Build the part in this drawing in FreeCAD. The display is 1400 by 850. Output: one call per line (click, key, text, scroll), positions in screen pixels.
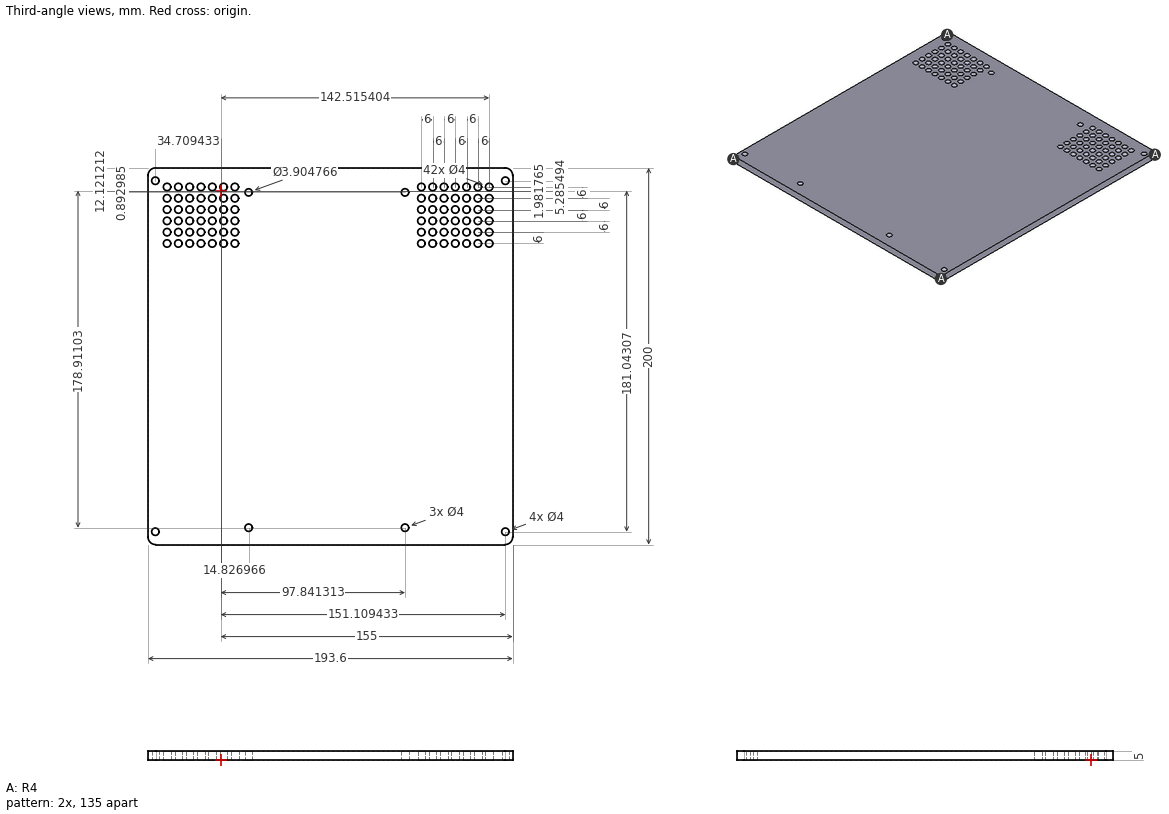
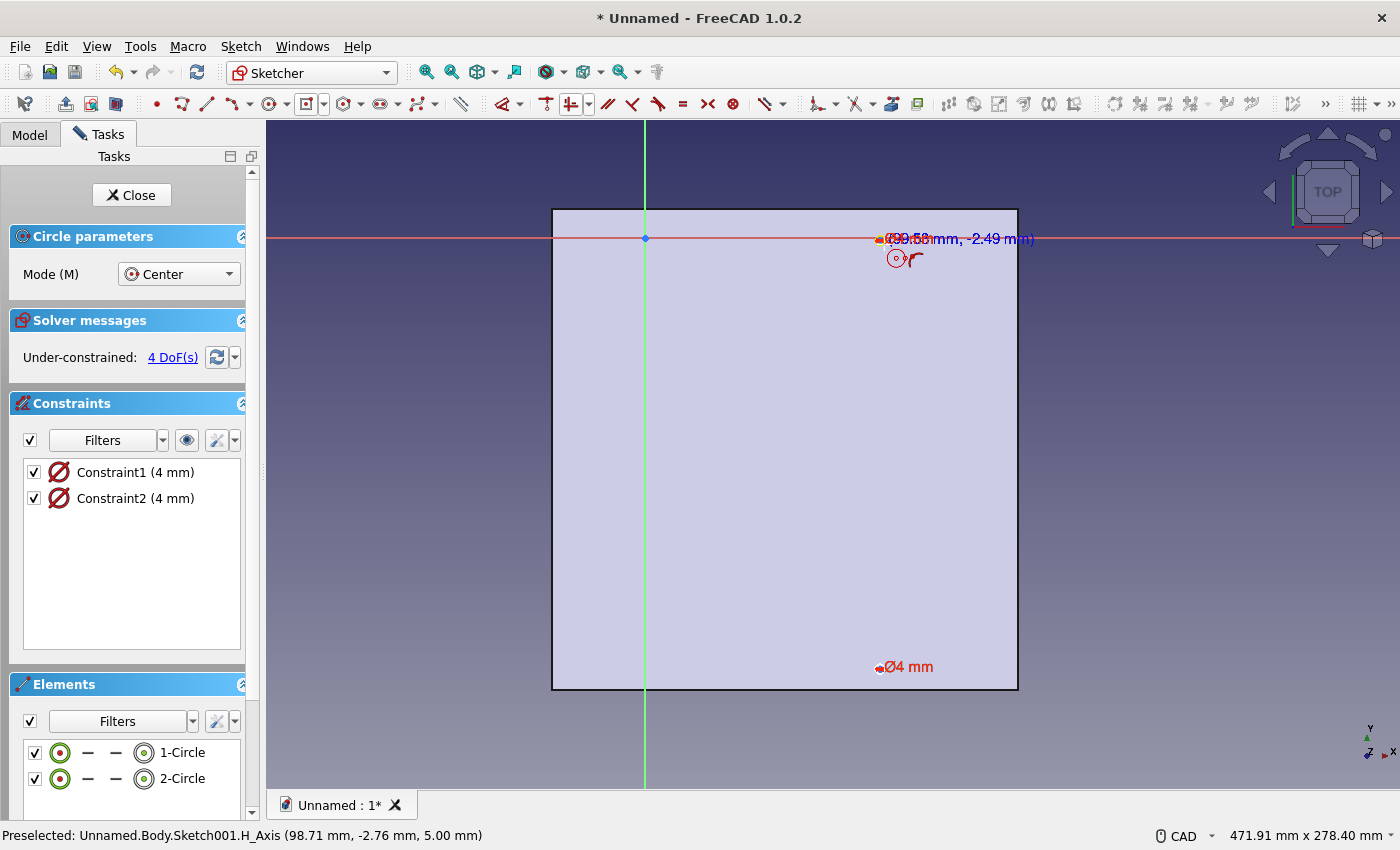
scroll(681, 668, up, 8)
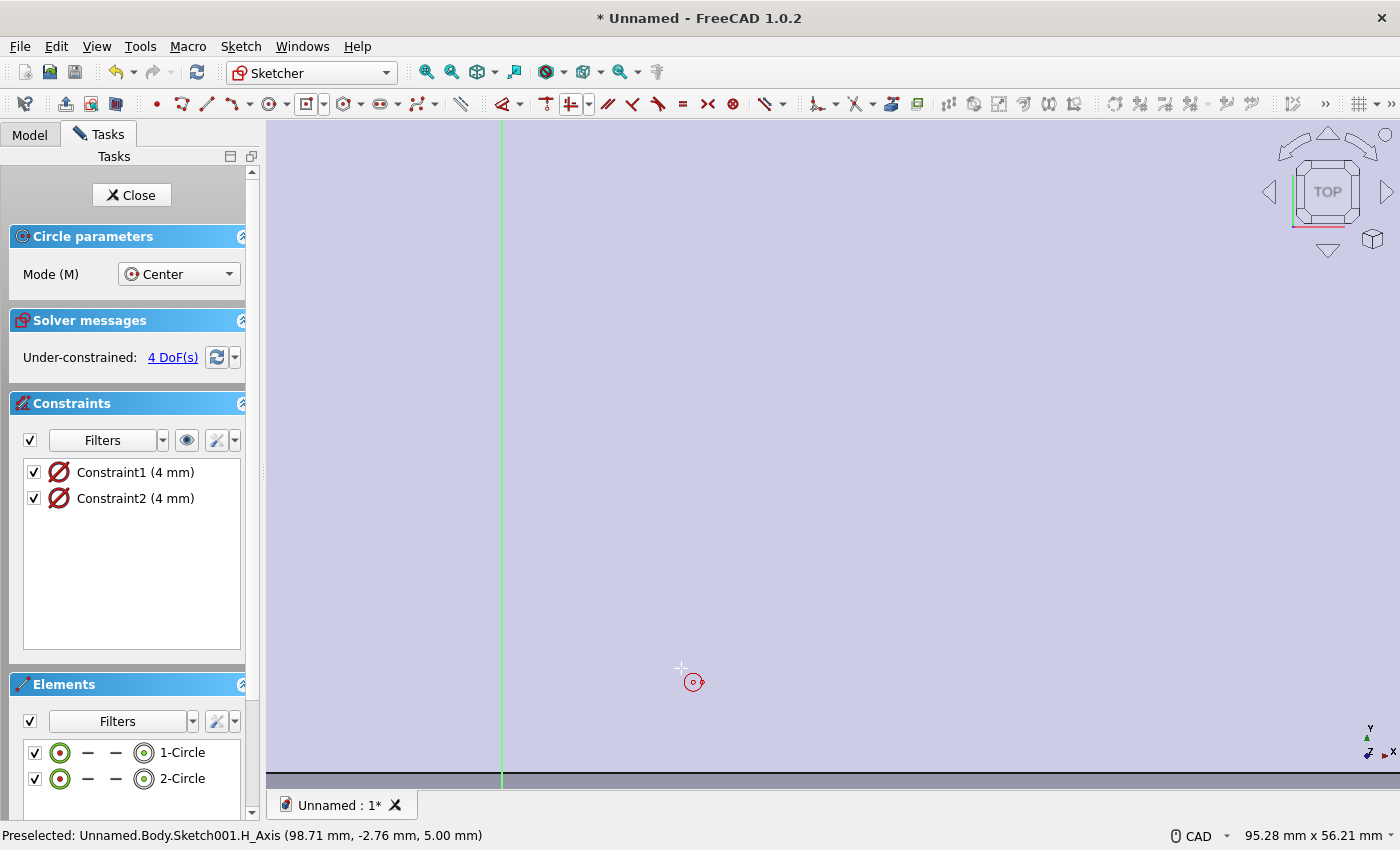
scroll(681, 669, down, 8)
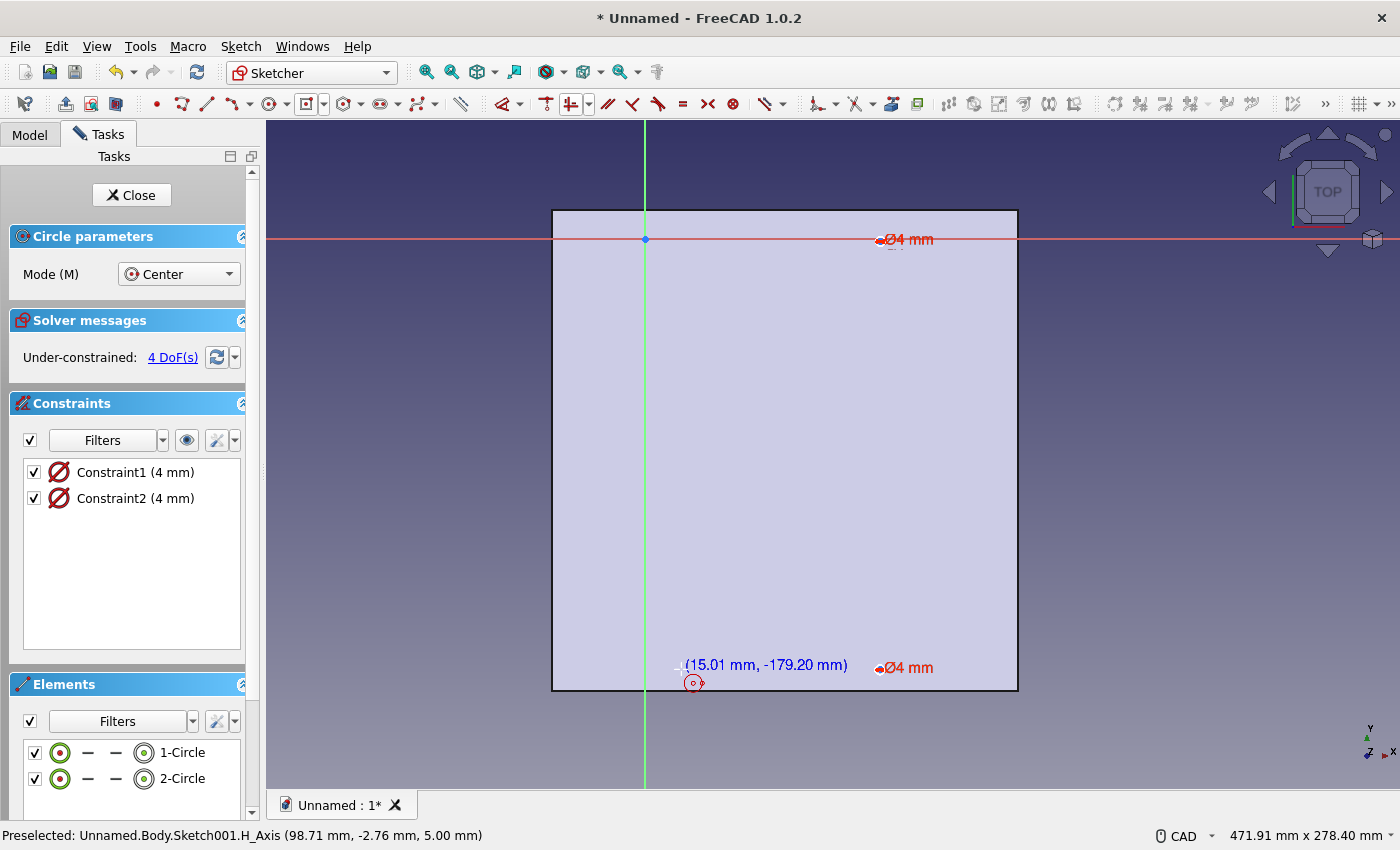
click(681, 669)
move(684, 666)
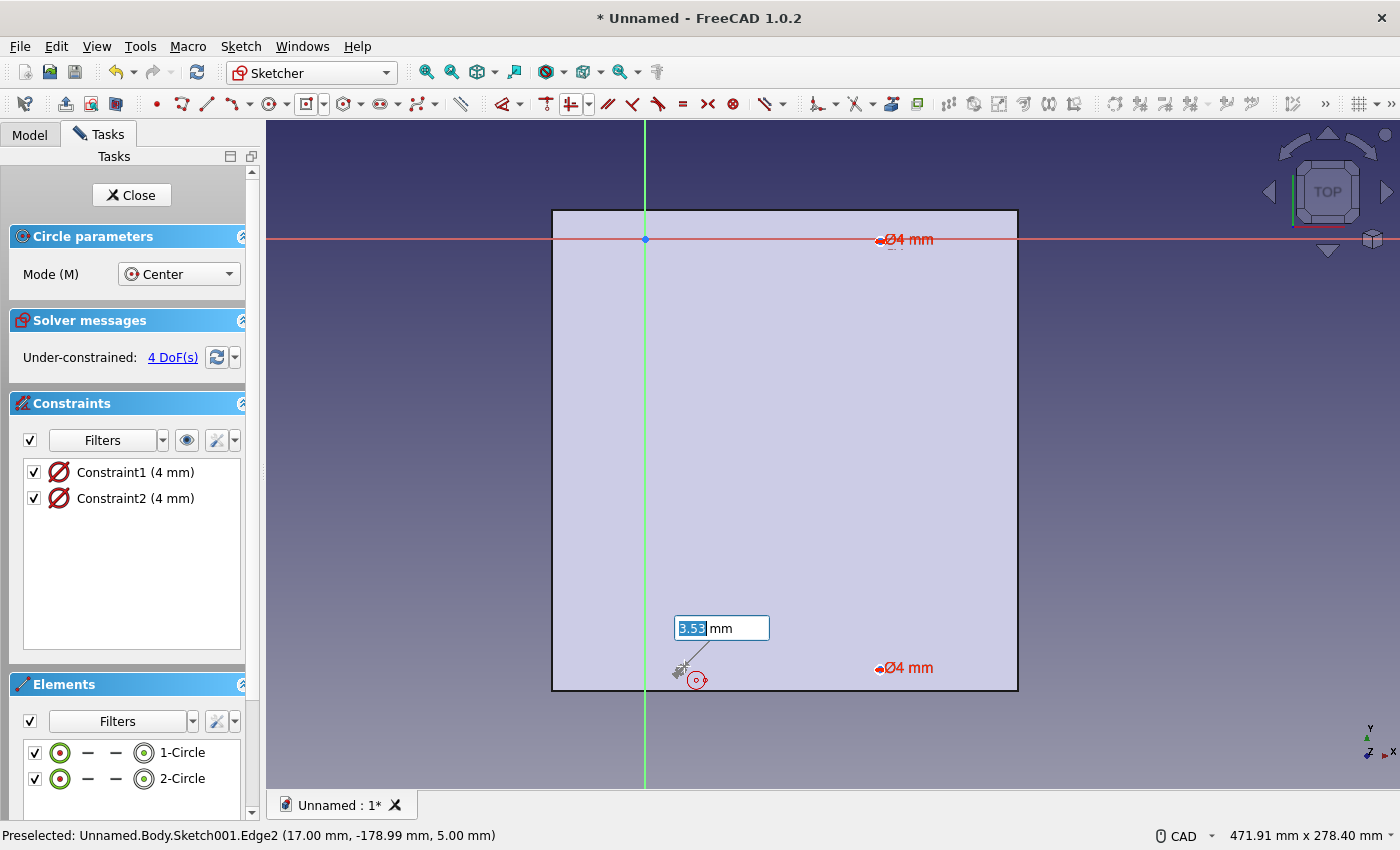
text(4)
key(Return)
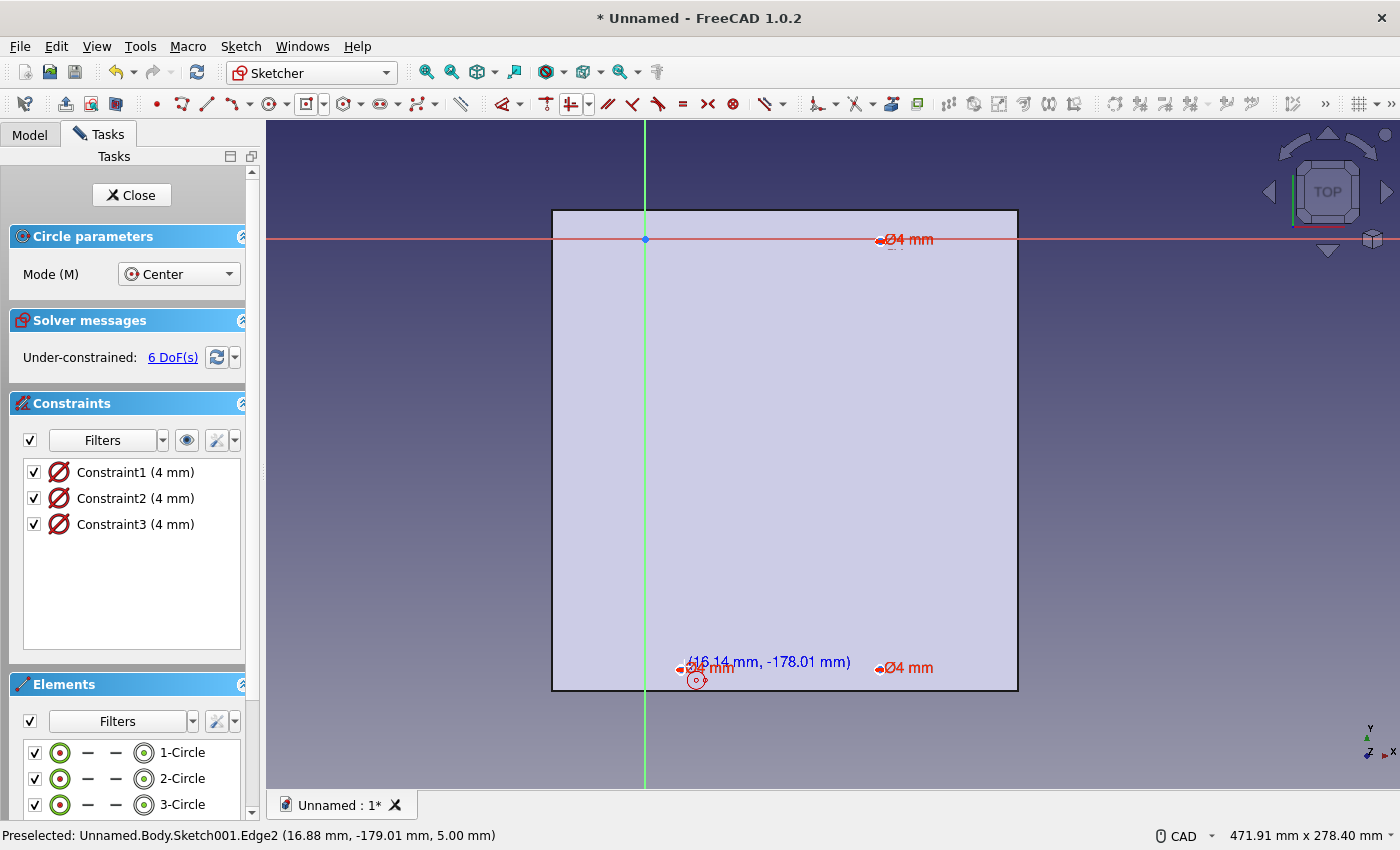
scroll(681, 241, up, 11)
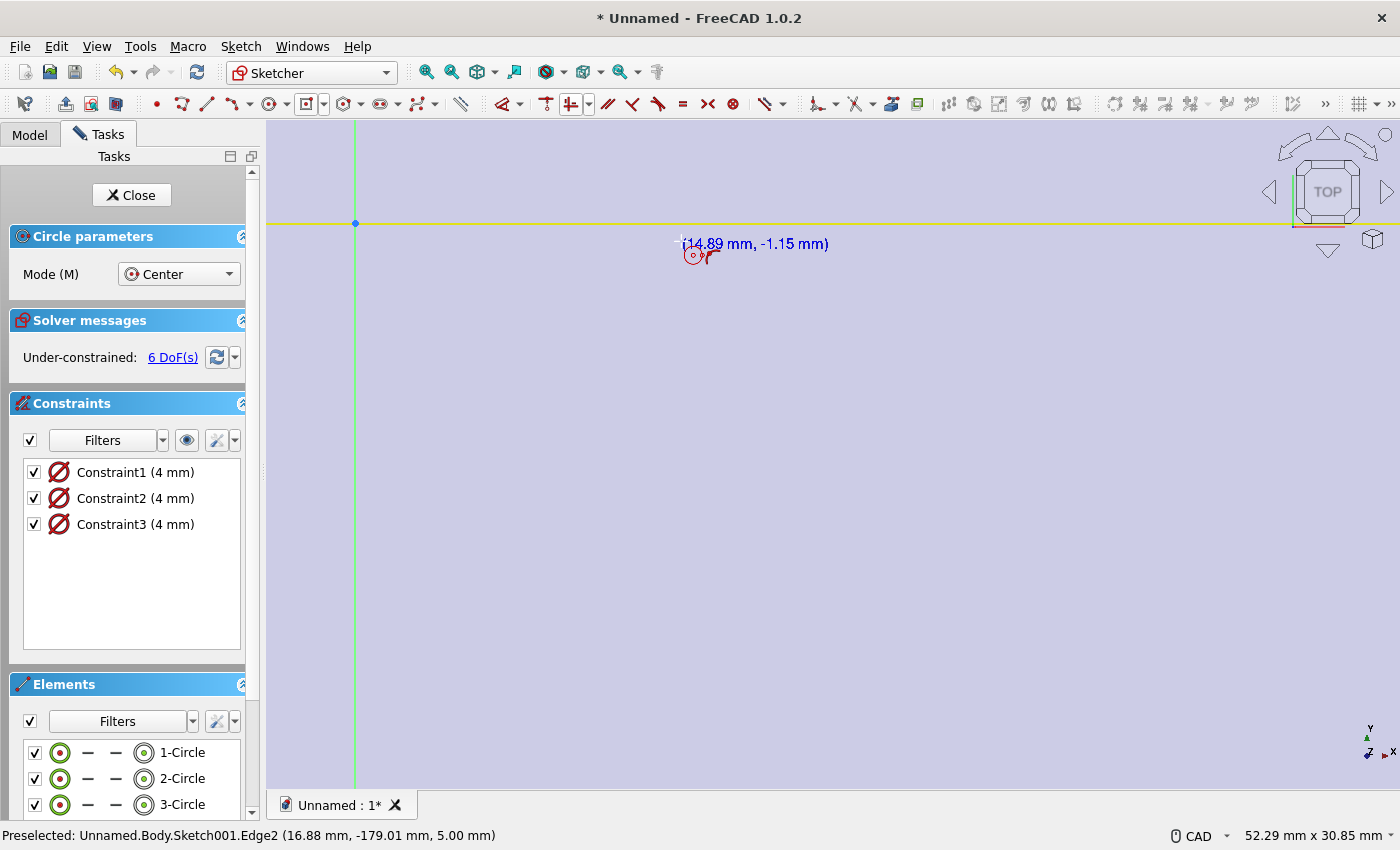
click(677, 243)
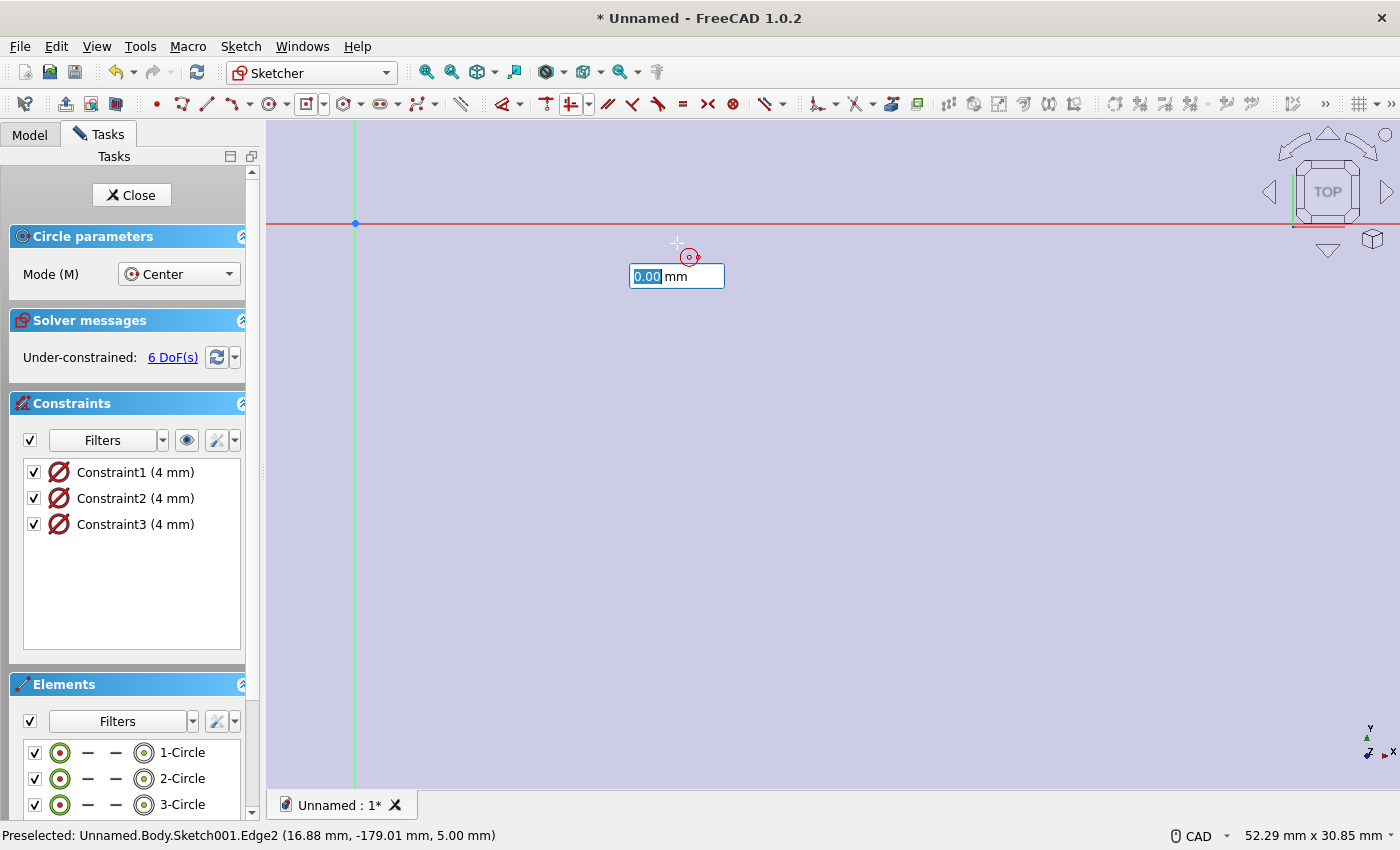
scroll(681, 240, down, 11)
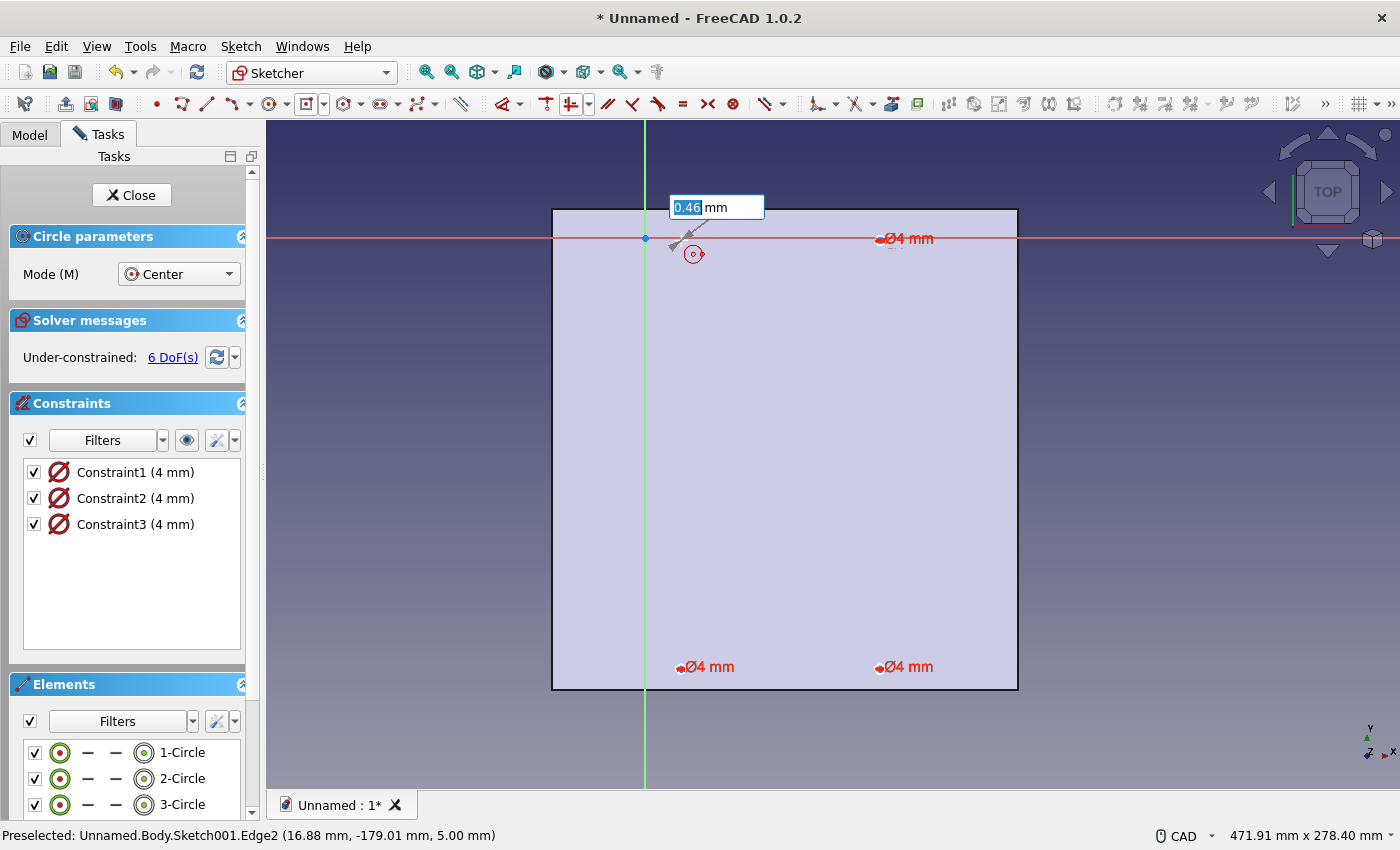
scroll(684, 244, up, 6)
move(684, 243)